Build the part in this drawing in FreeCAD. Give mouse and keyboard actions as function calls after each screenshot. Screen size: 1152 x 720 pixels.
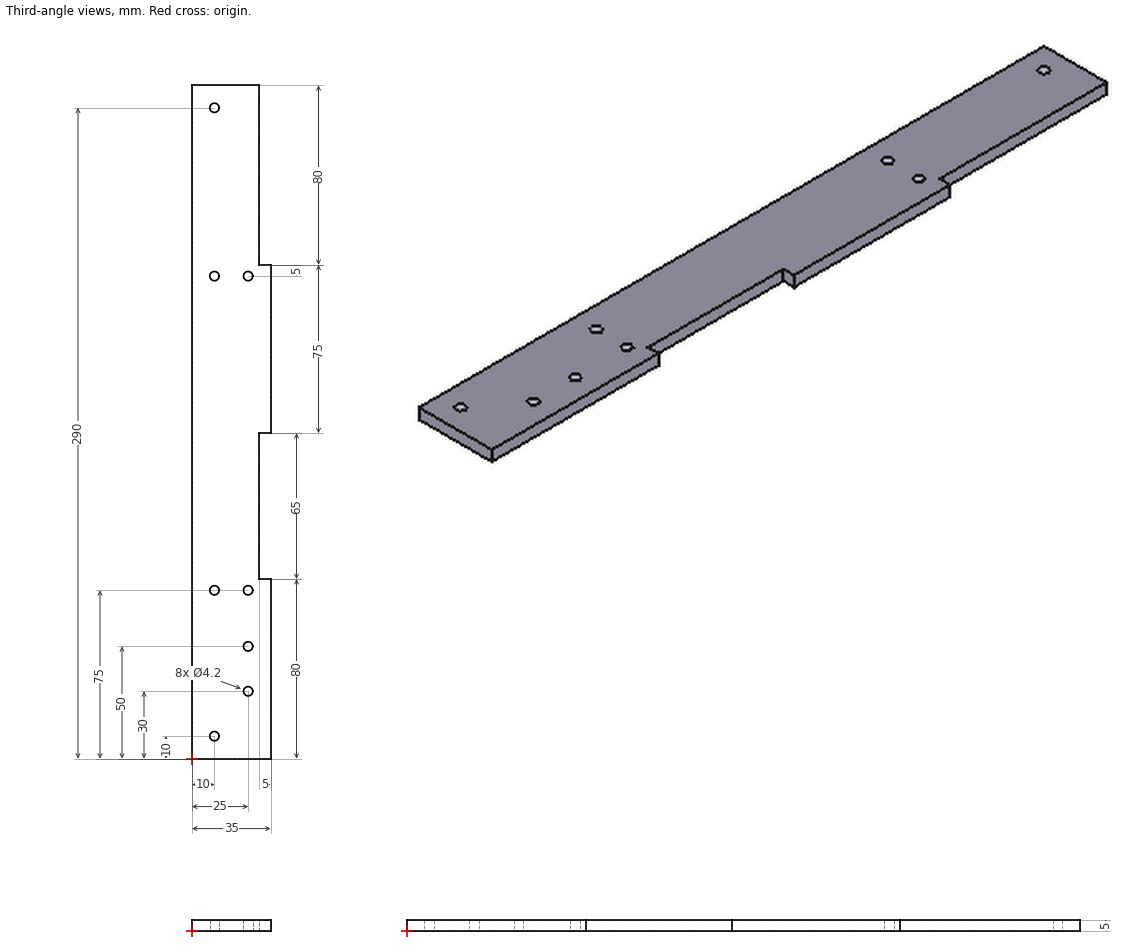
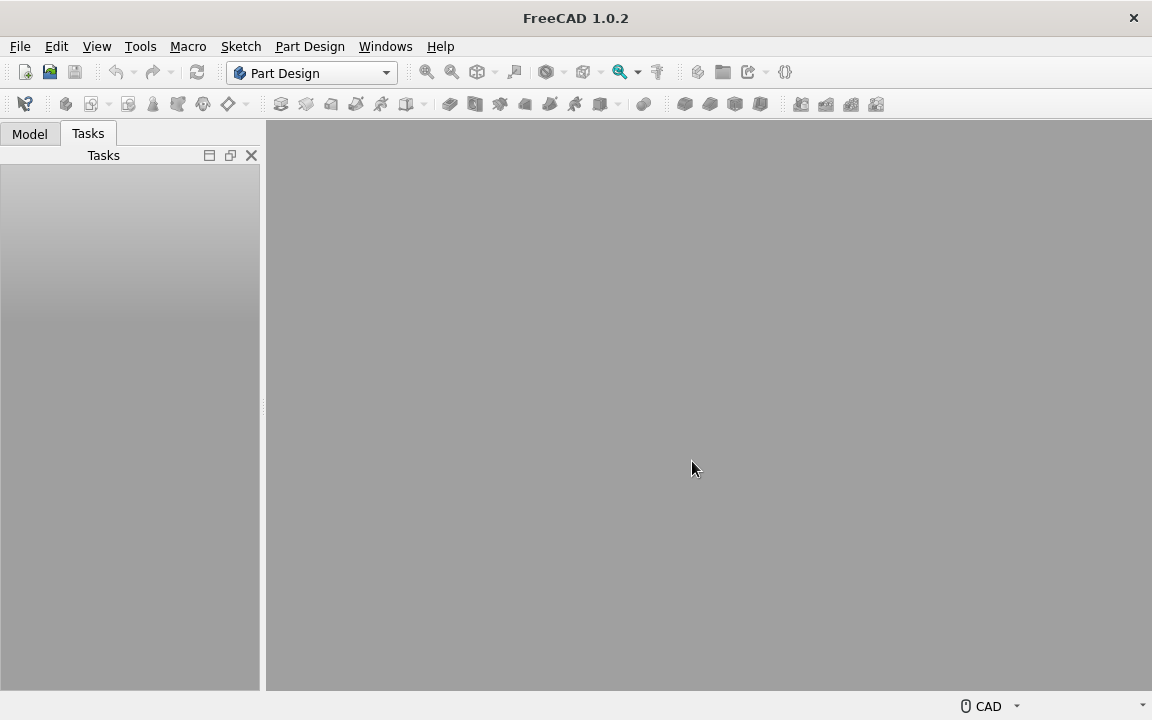
click(25, 72)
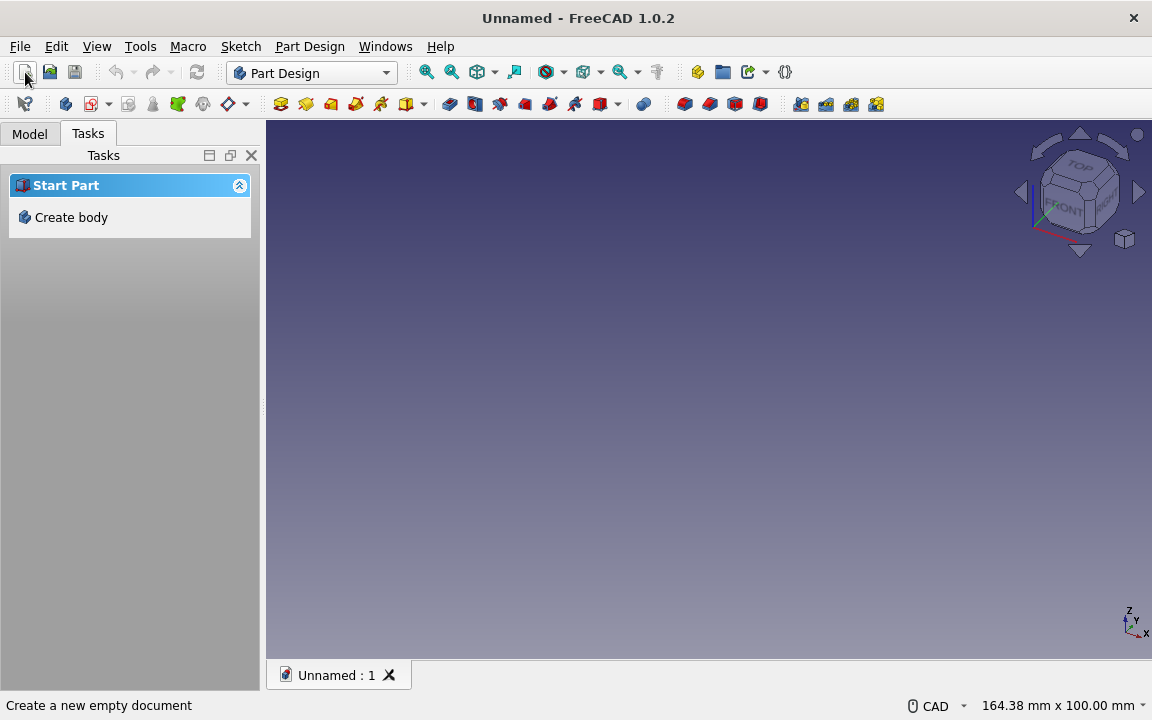
click(90, 104)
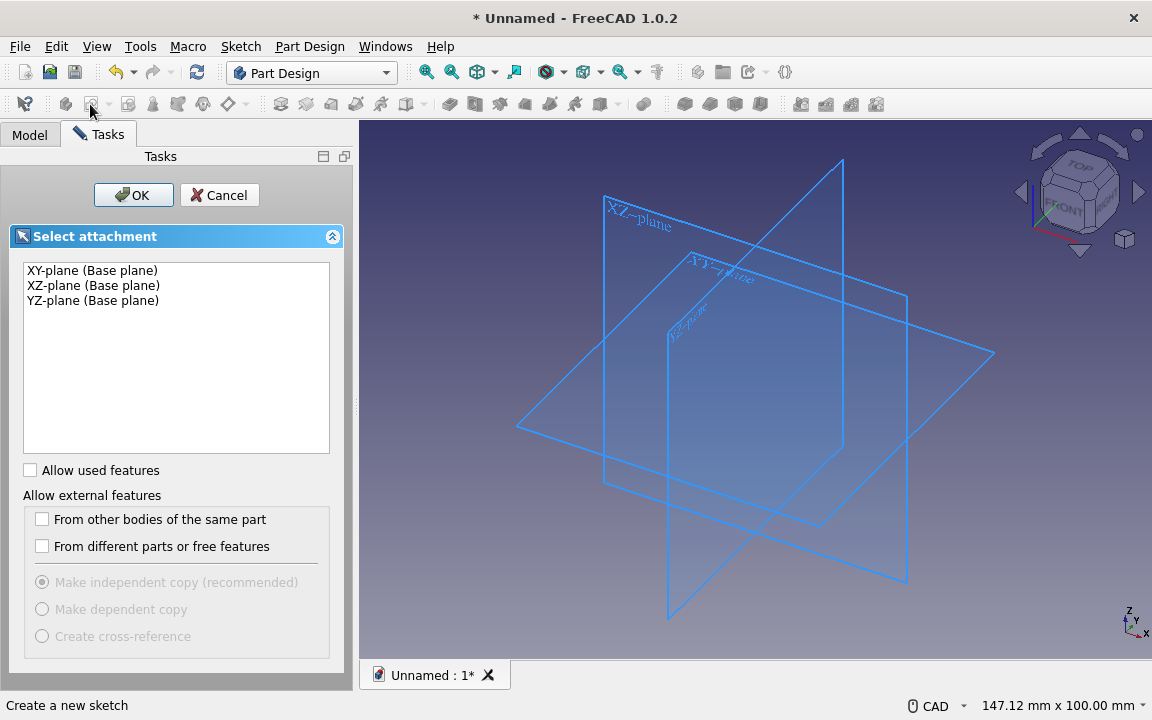
click(84, 270)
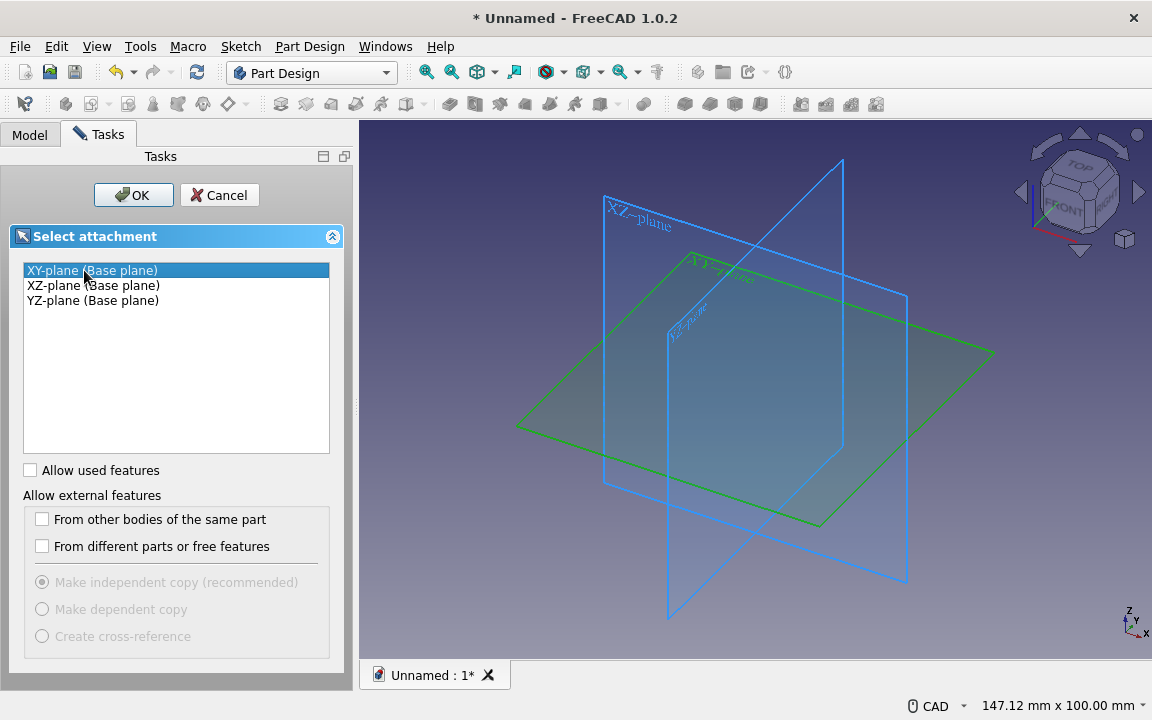
click(134, 195)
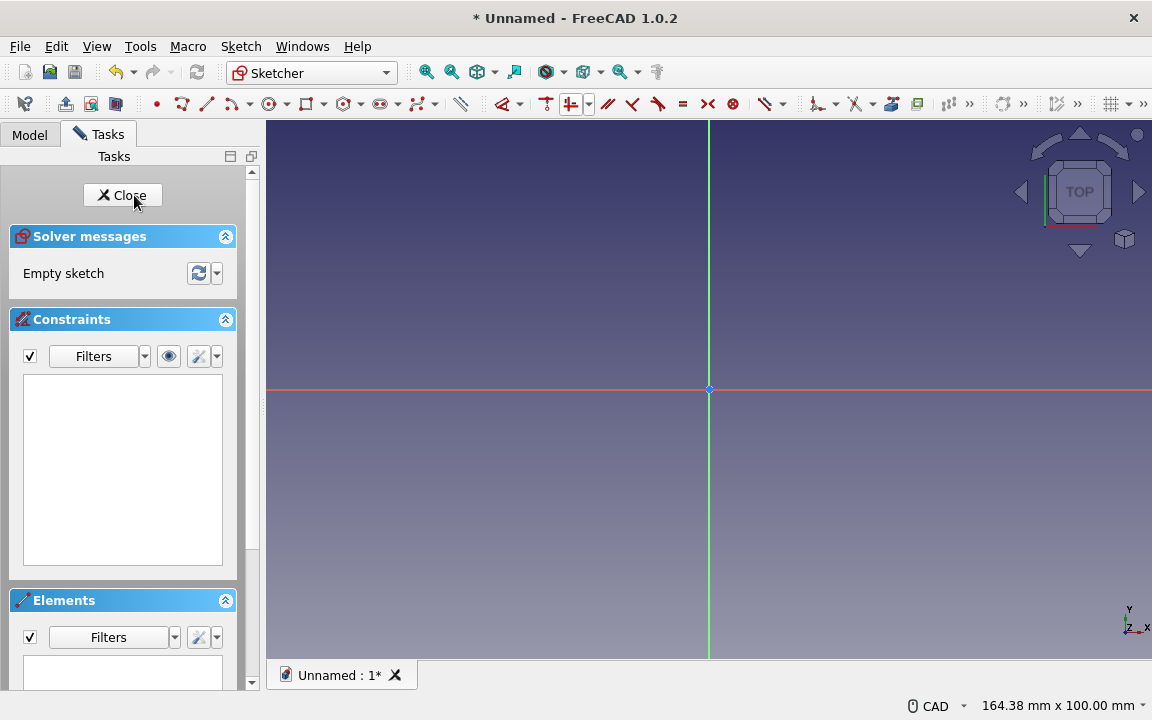
scroll(599, 594, down, 8)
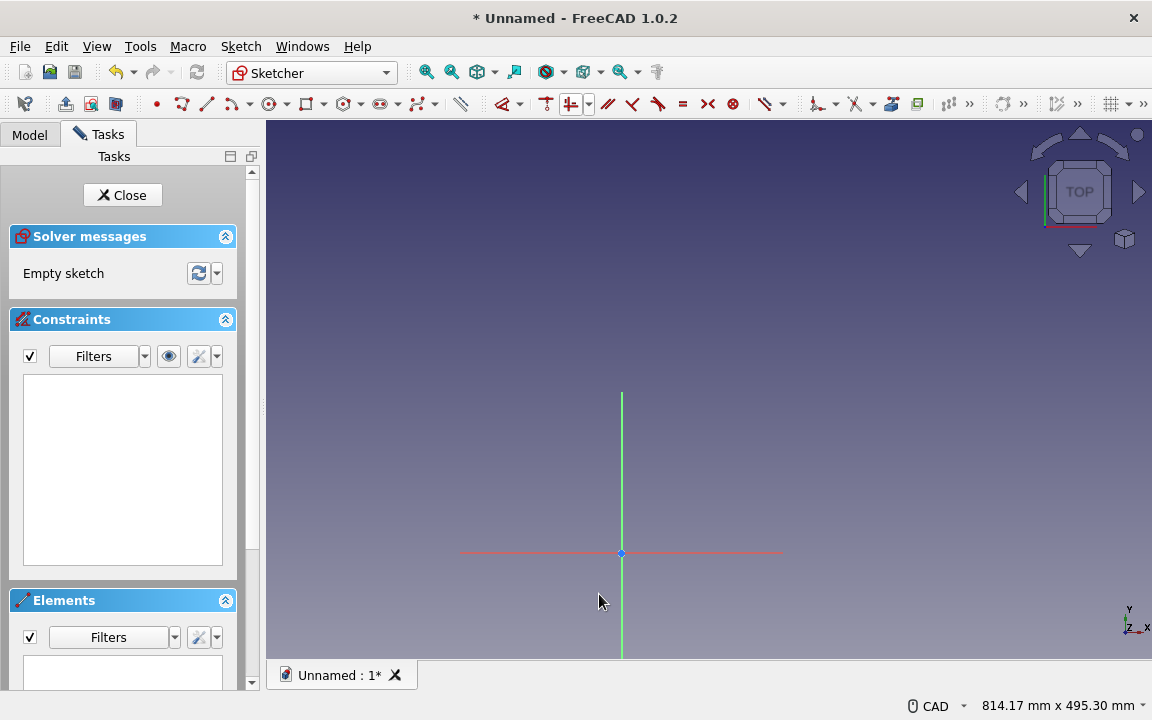
click(182, 104)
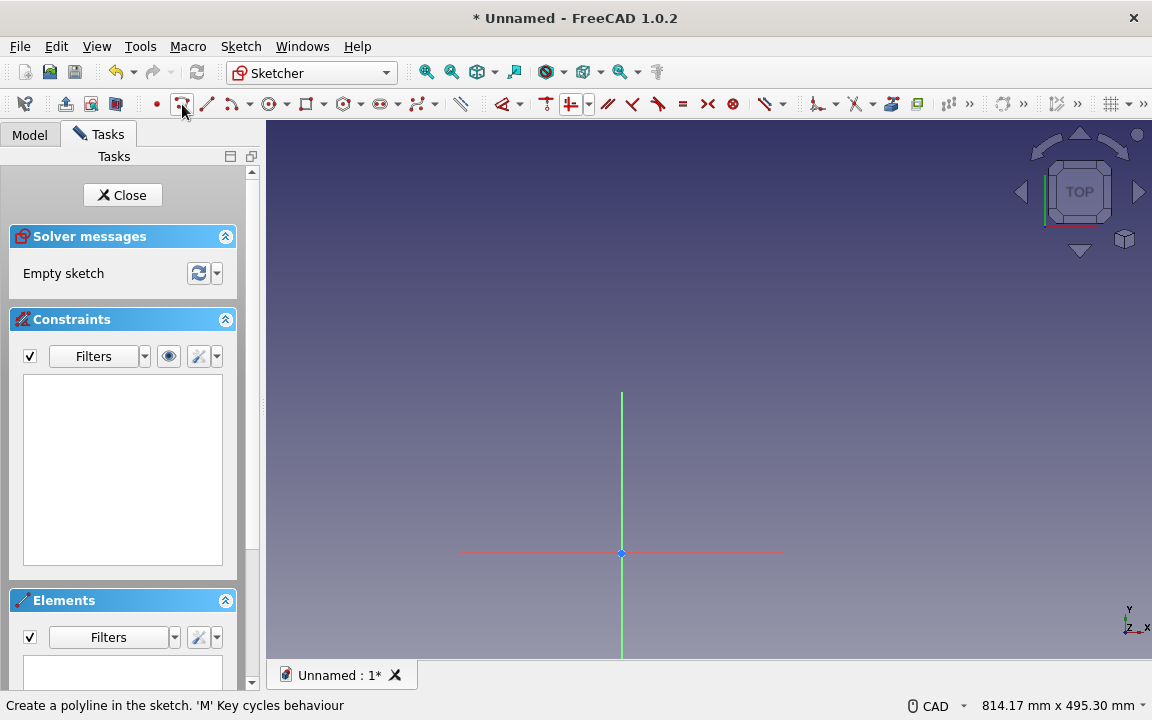
click(622, 553)
click(660, 544)
click(660, 466)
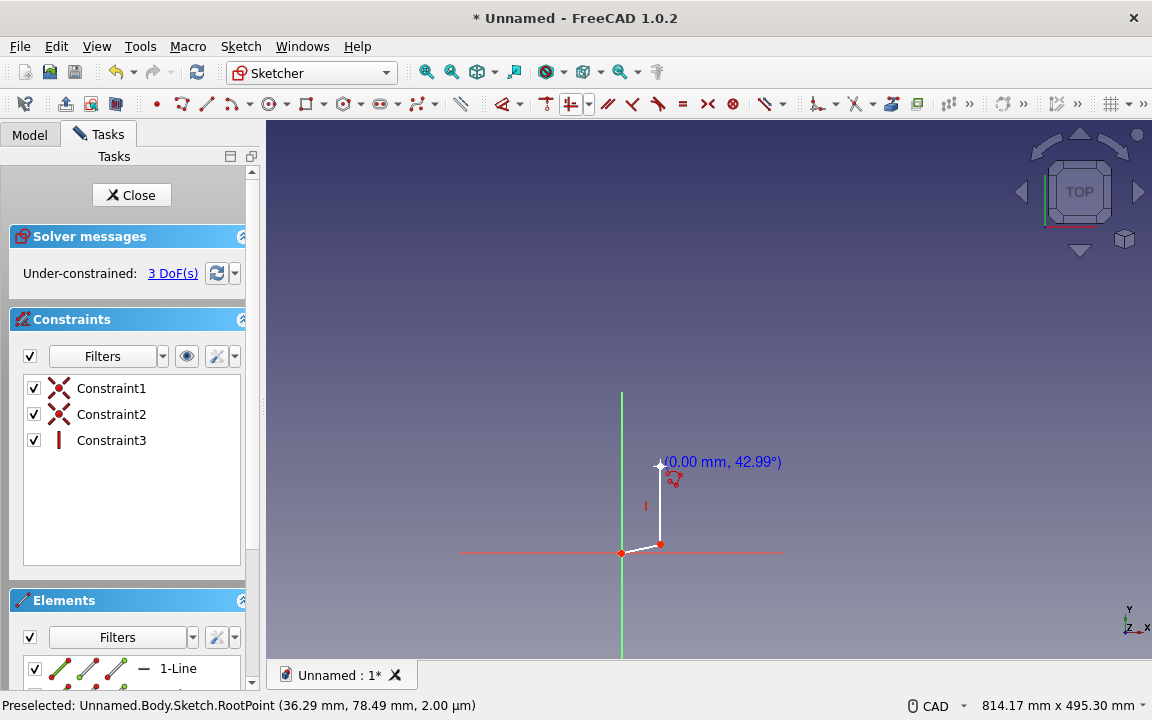
scroll(654, 466, up, 6)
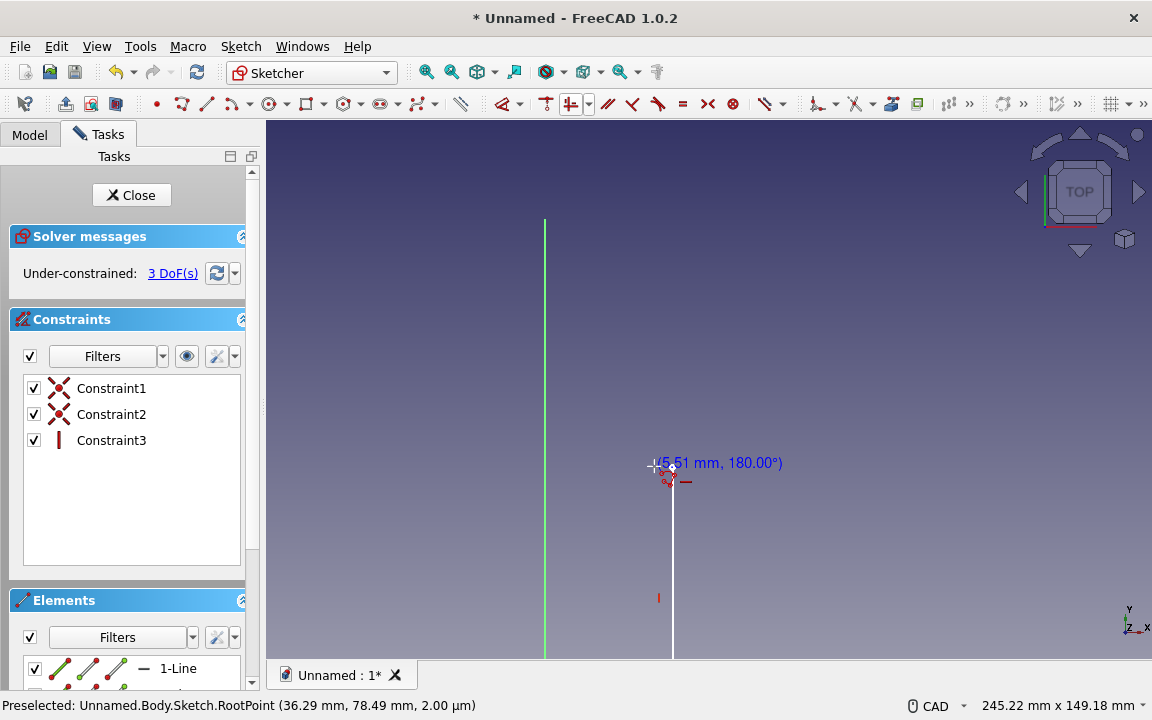
click(653, 465)
click(653, 231)
click(672, 231)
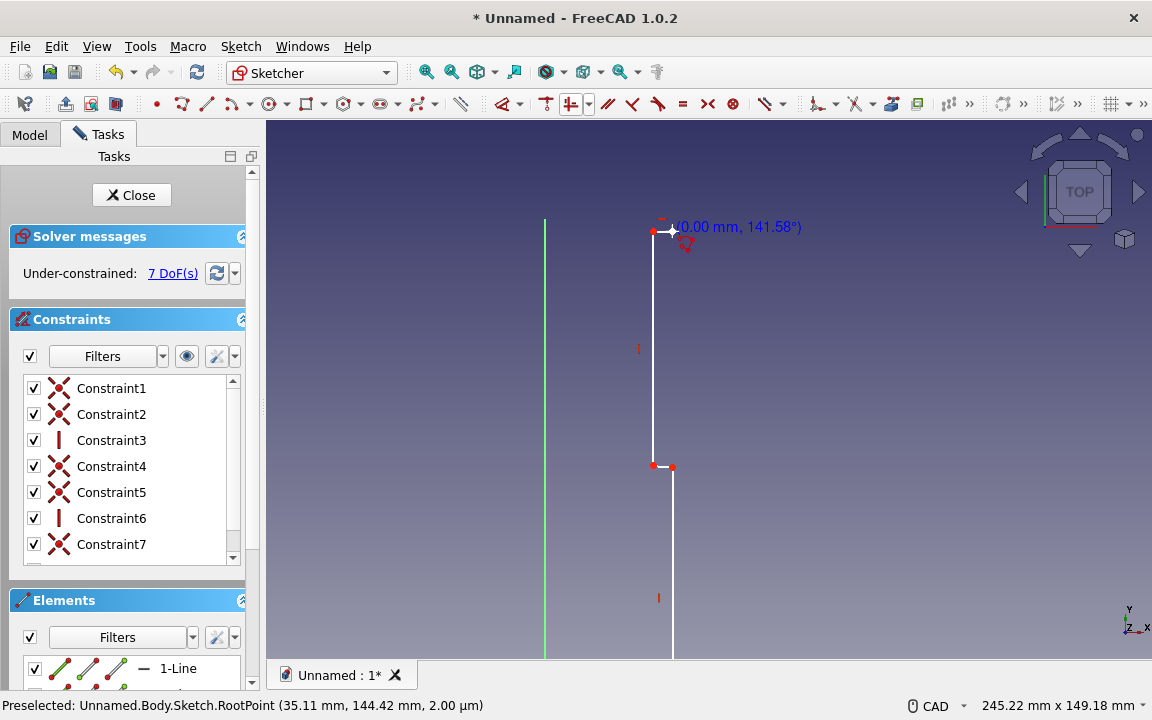
scroll(654, 466, down, 6)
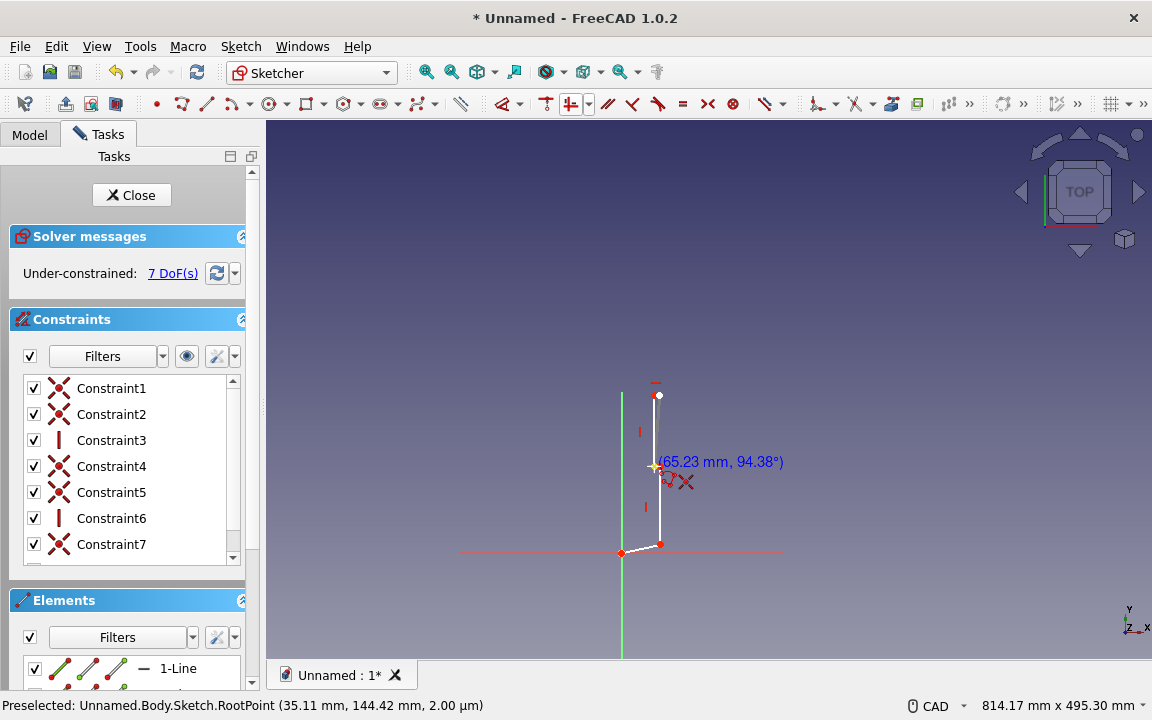
click(660, 314)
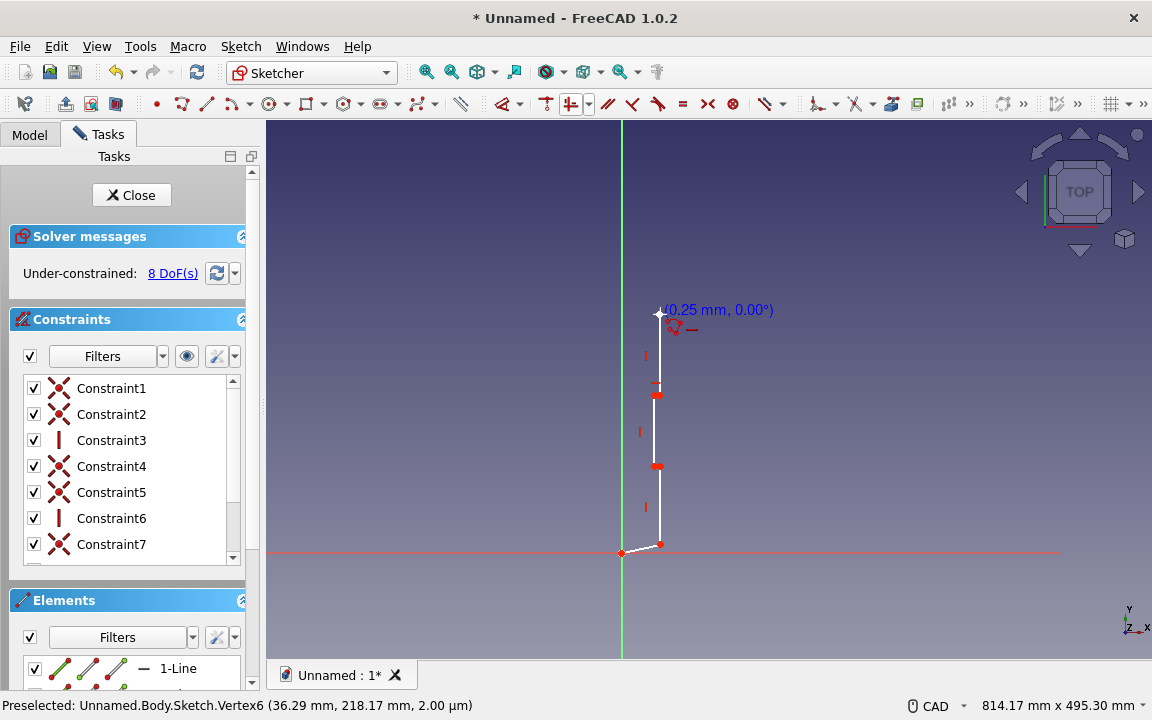
scroll(654, 314, up, 6)